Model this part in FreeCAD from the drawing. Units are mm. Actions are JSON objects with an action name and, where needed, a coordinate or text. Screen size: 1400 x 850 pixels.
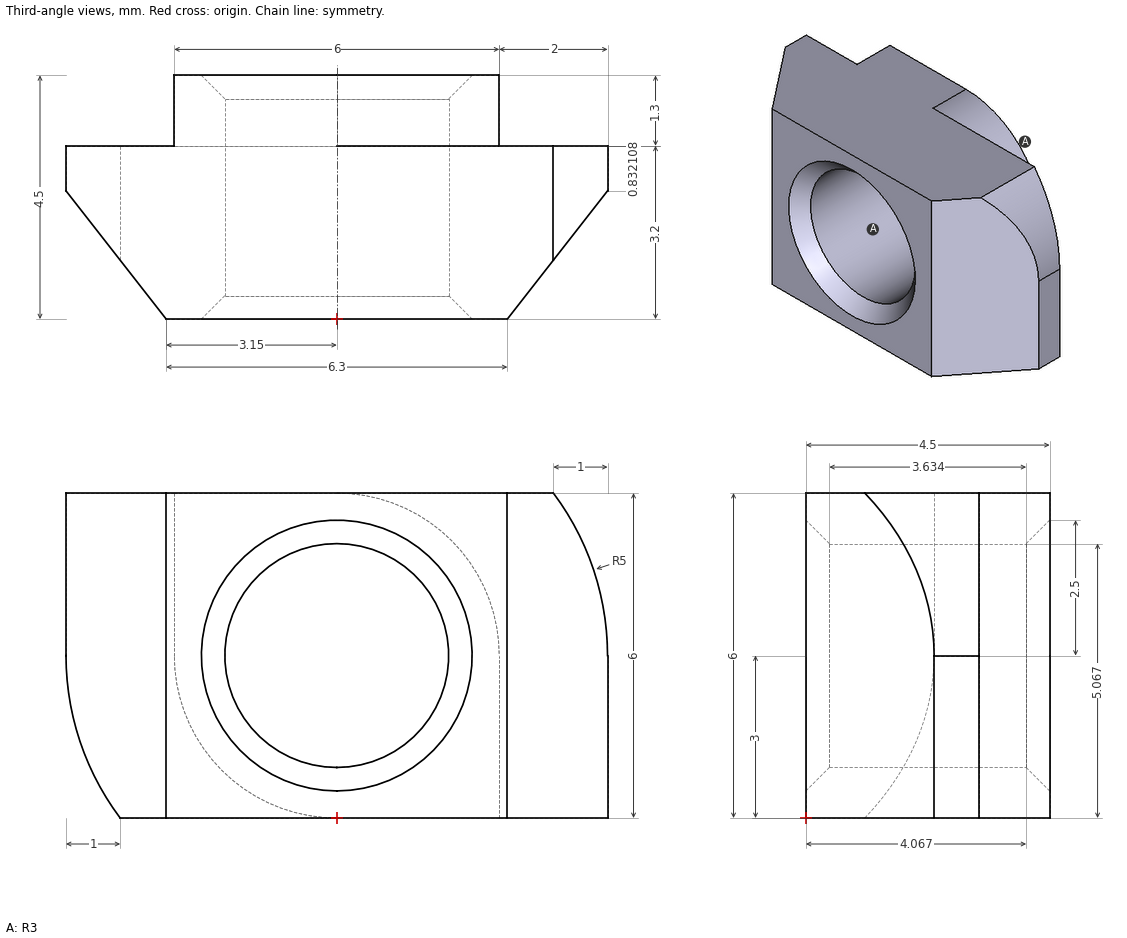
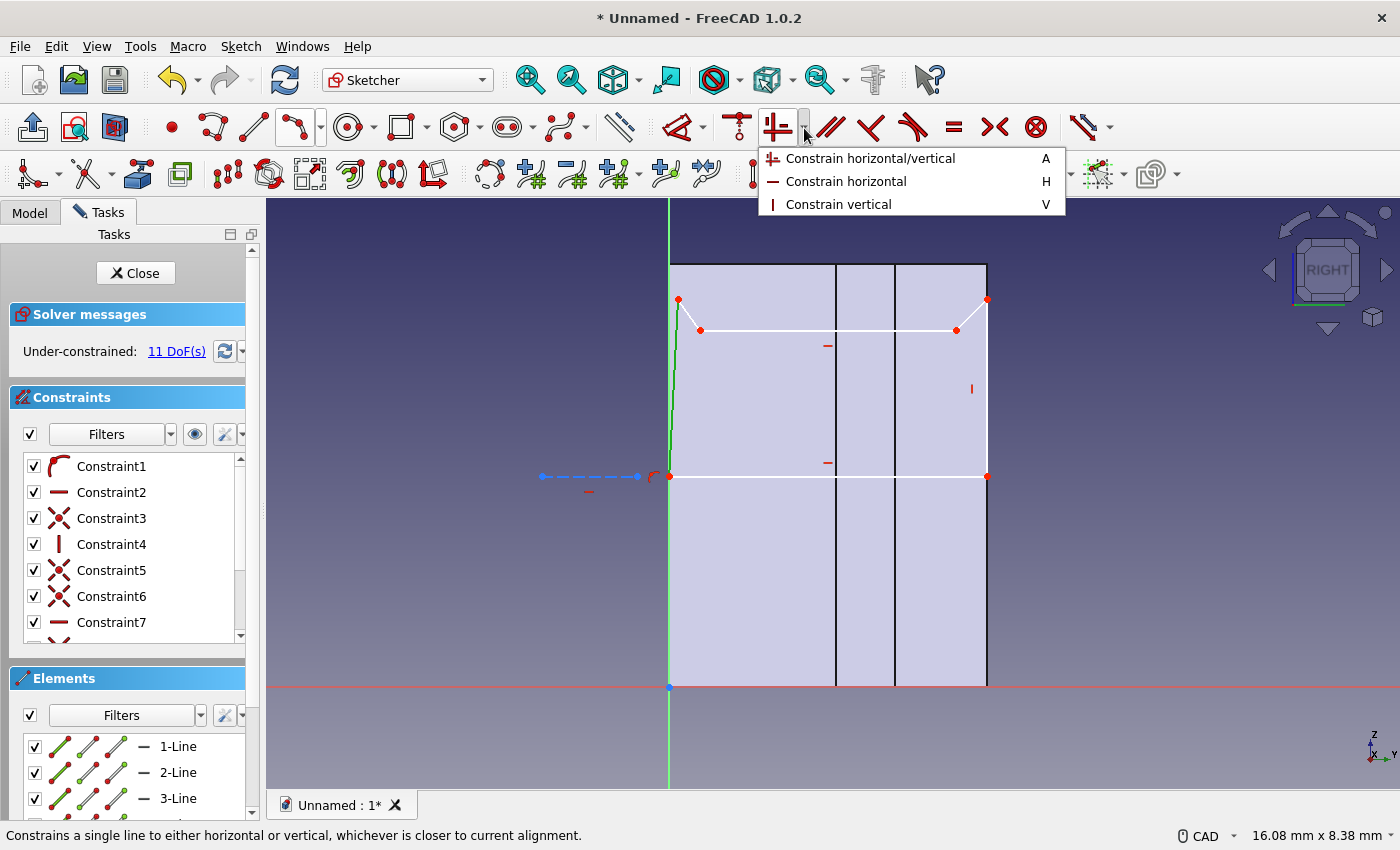
{"action": "left_click", "coordinate": [912, 204]}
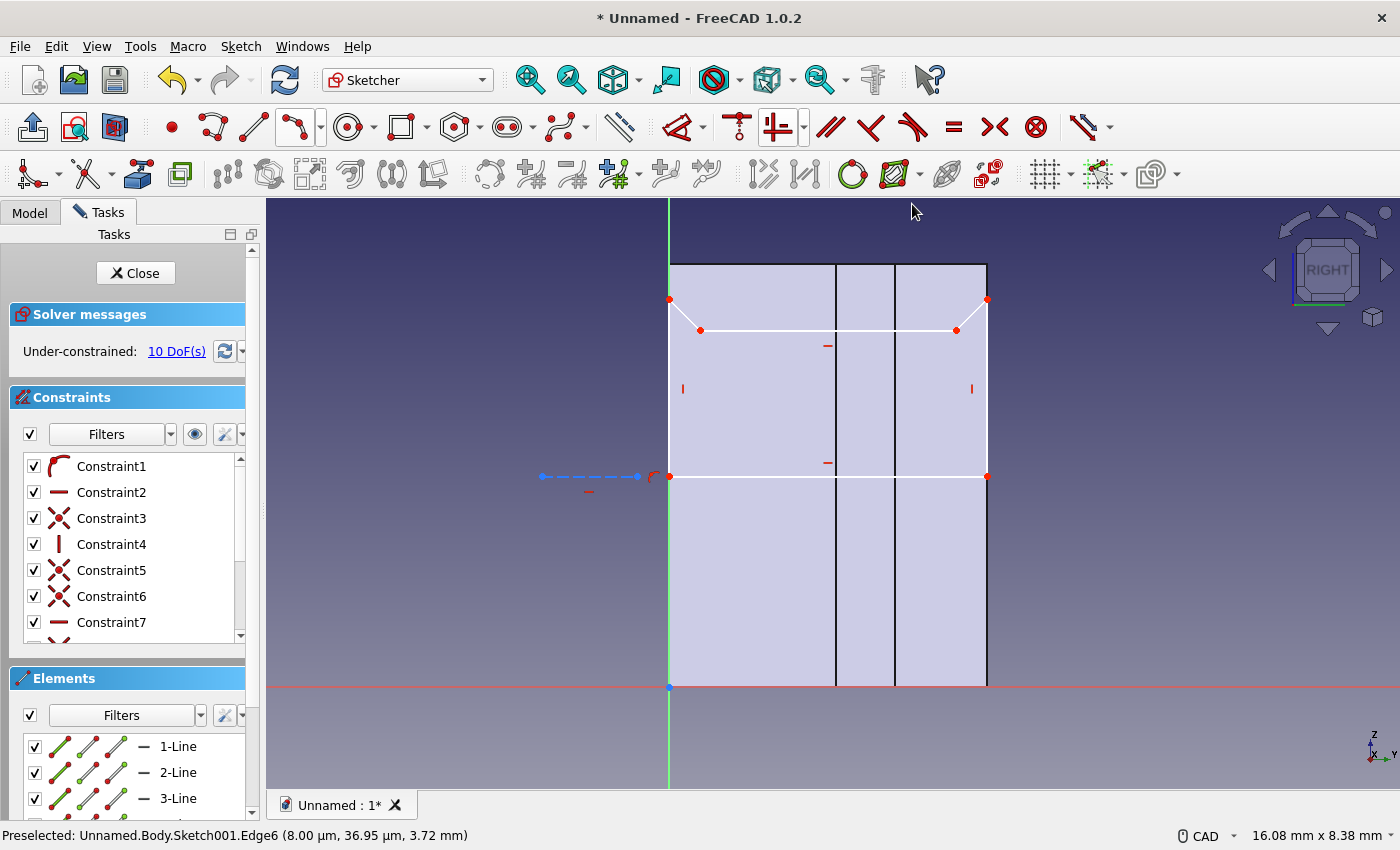
{"action": "left_click", "coordinate": [676, 128]}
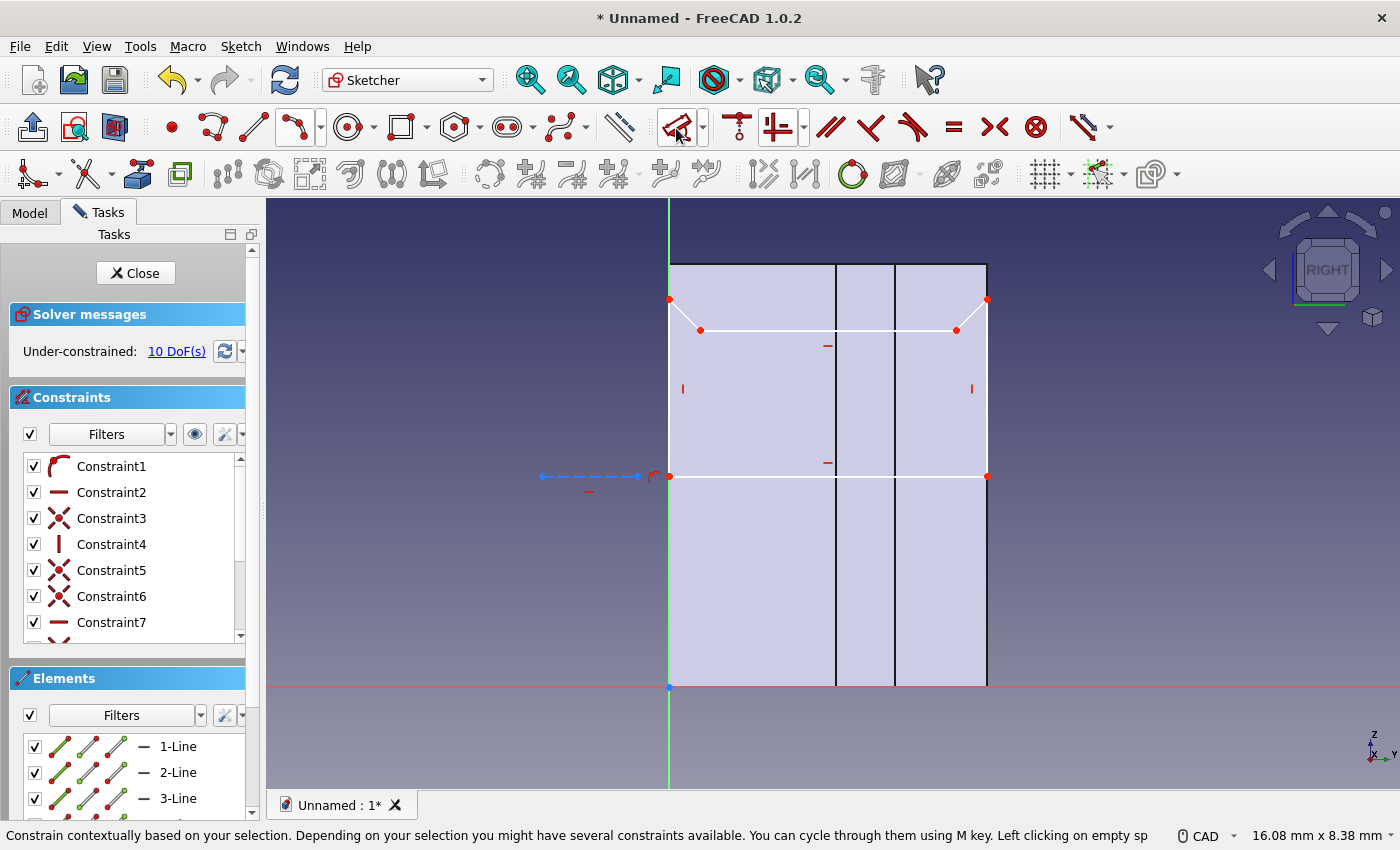
{"action": "left_click", "coordinate": [669, 477]}
{"action": "left_click", "coordinate": [635, 582]}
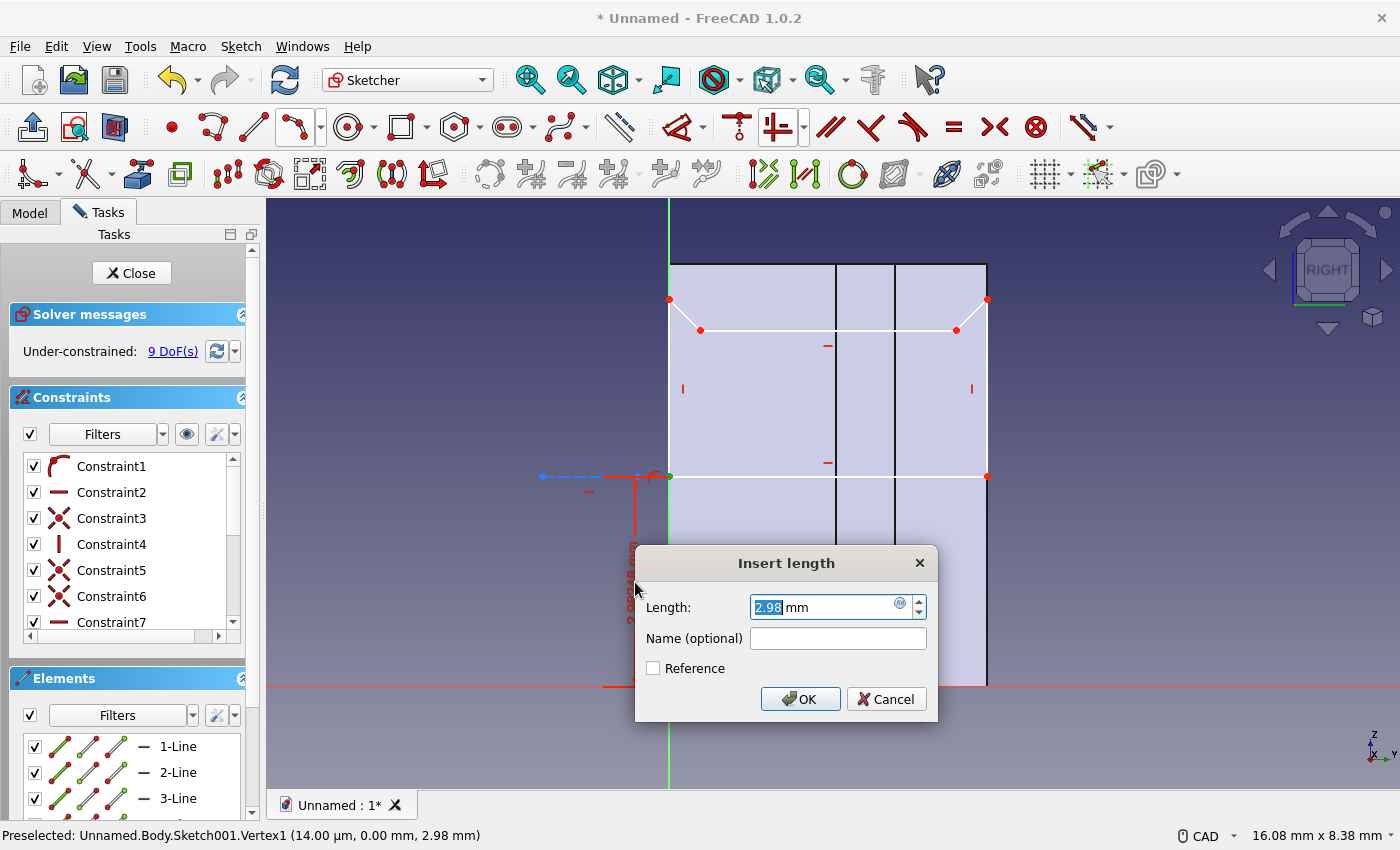
{"action": "type", "text": "3"}
{"action": "key", "text": "Return"}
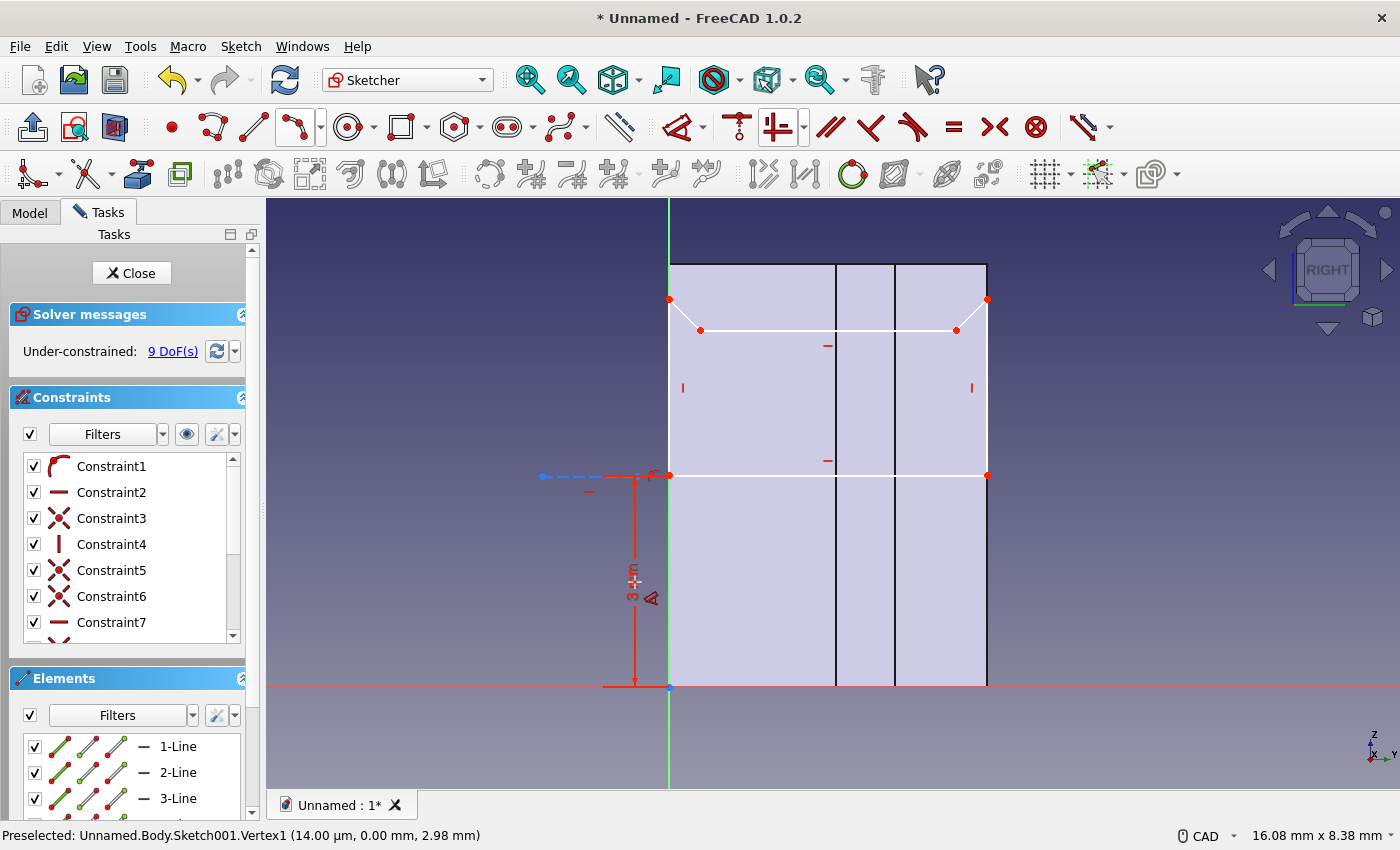
{"action": "left_click", "coordinate": [637, 477]}
{"action": "left_click", "coordinate": [603, 534]}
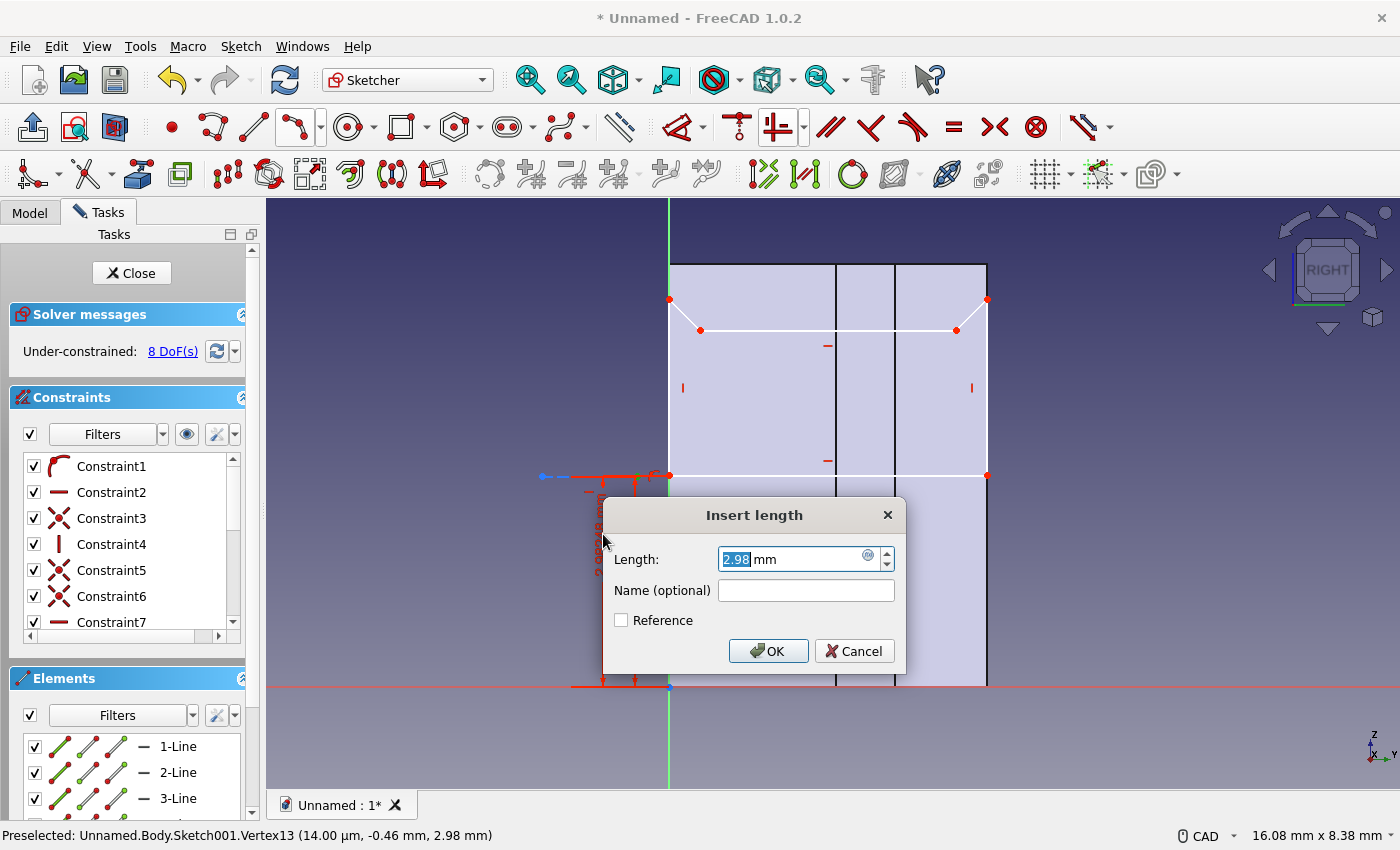
{"action": "type", "text": "3"}
{"action": "key", "text": "Return"}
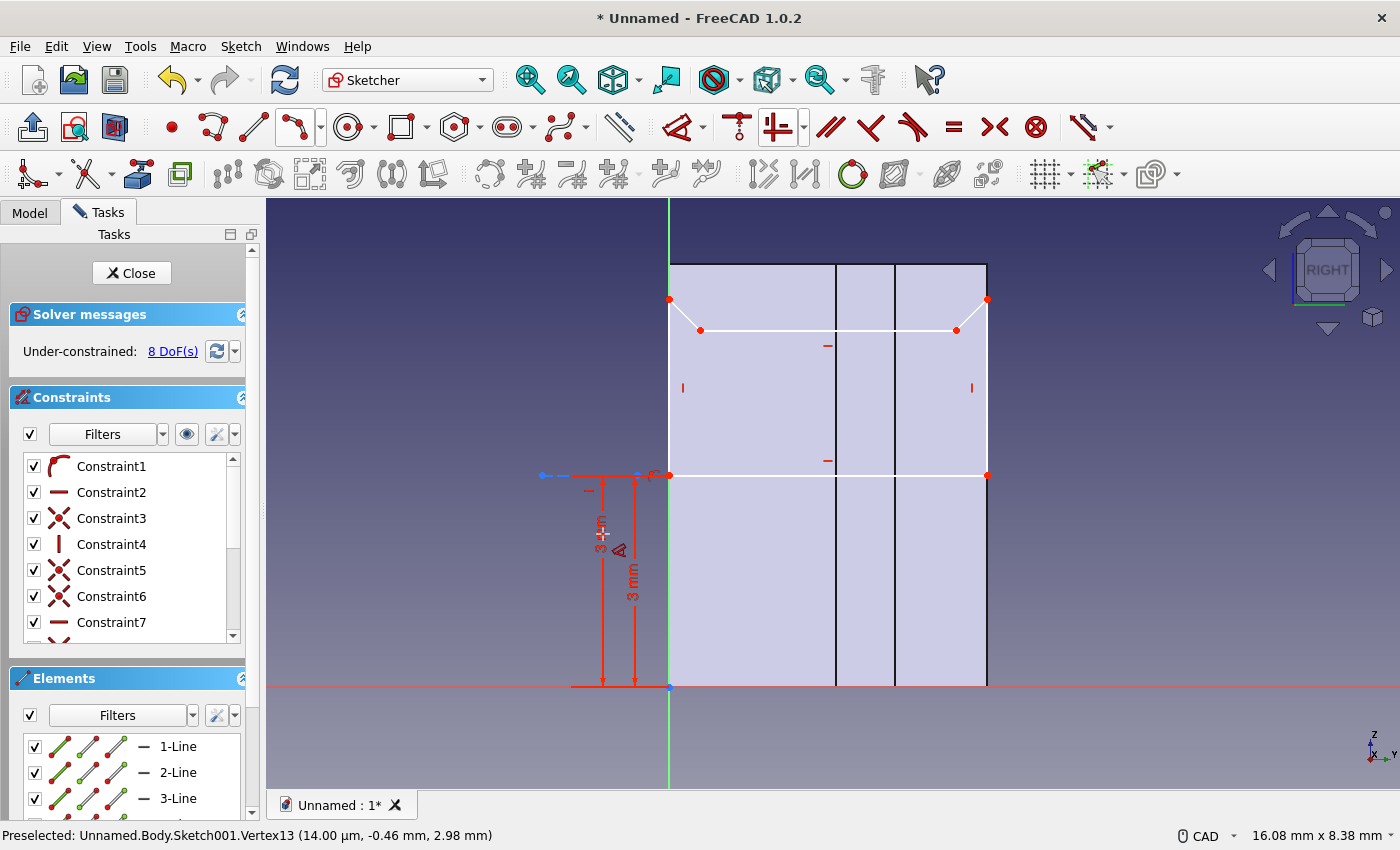
{"action": "left_click", "coordinate": [764, 476]}
{"action": "left_click", "coordinate": [828, 442]}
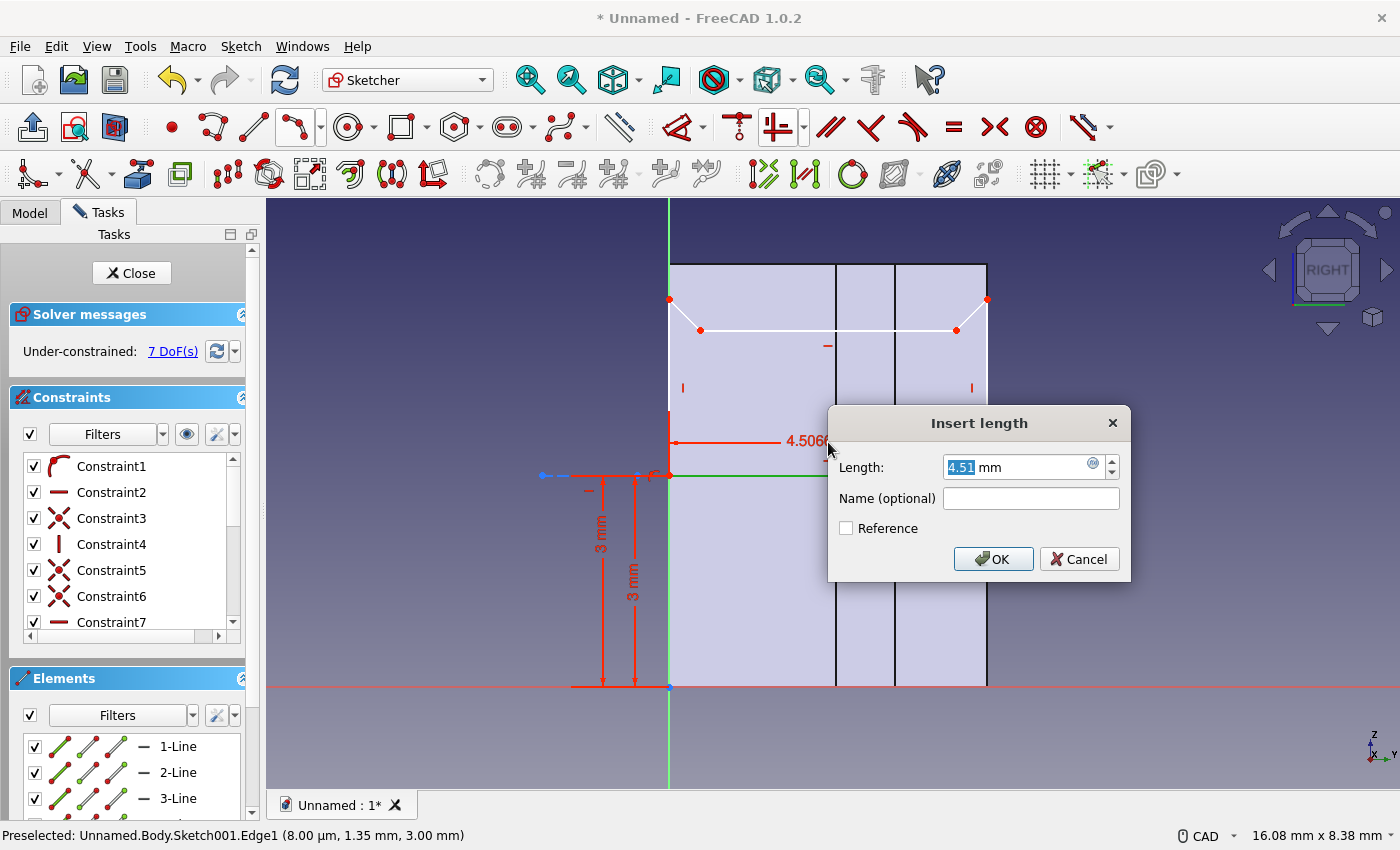
{"action": "type", "text": "4.5"}
{"action": "key", "text": "Return"}